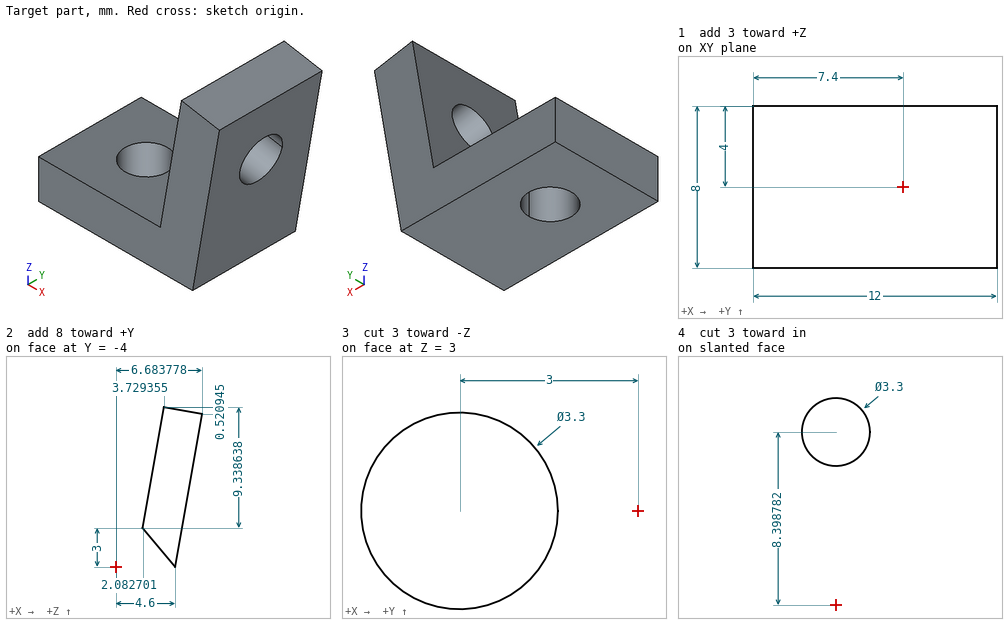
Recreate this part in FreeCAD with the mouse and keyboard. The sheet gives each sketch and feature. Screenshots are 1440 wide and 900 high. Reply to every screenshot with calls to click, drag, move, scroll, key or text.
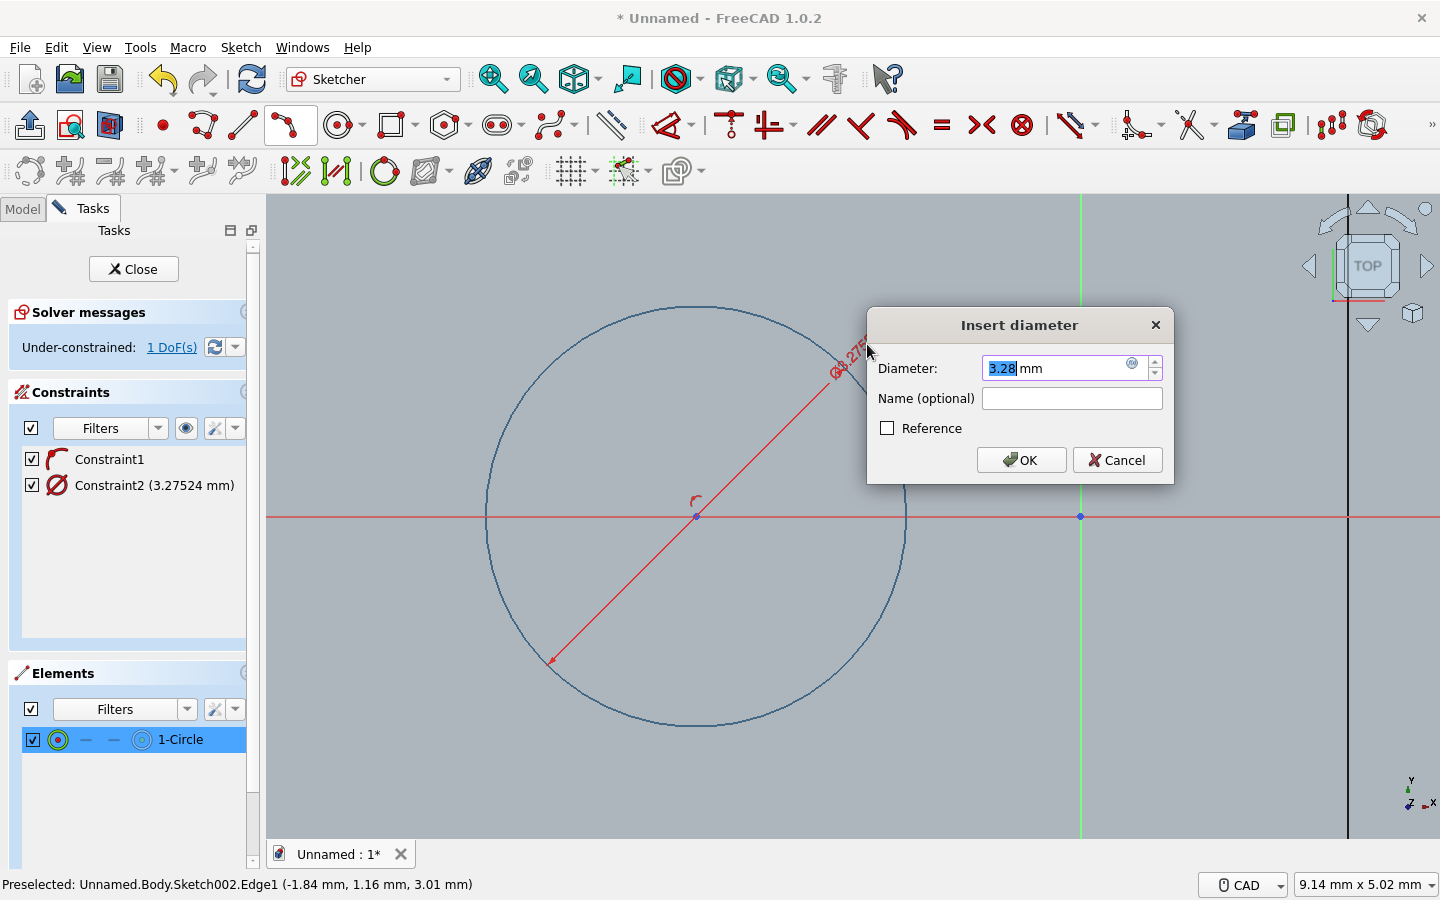
text(3.3)
key(Return)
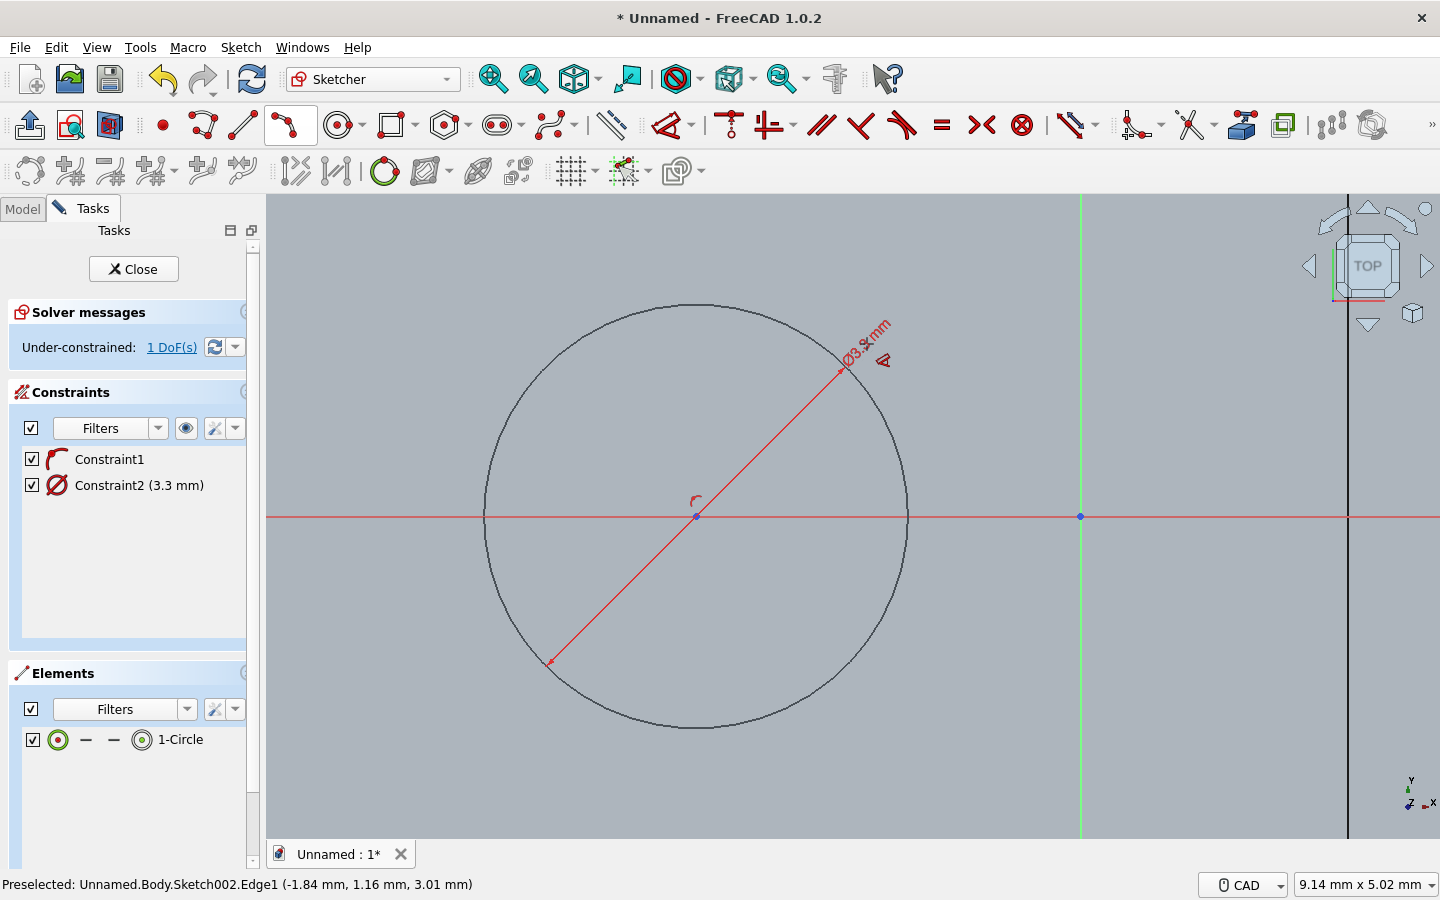
click(696, 516)
click(888, 550)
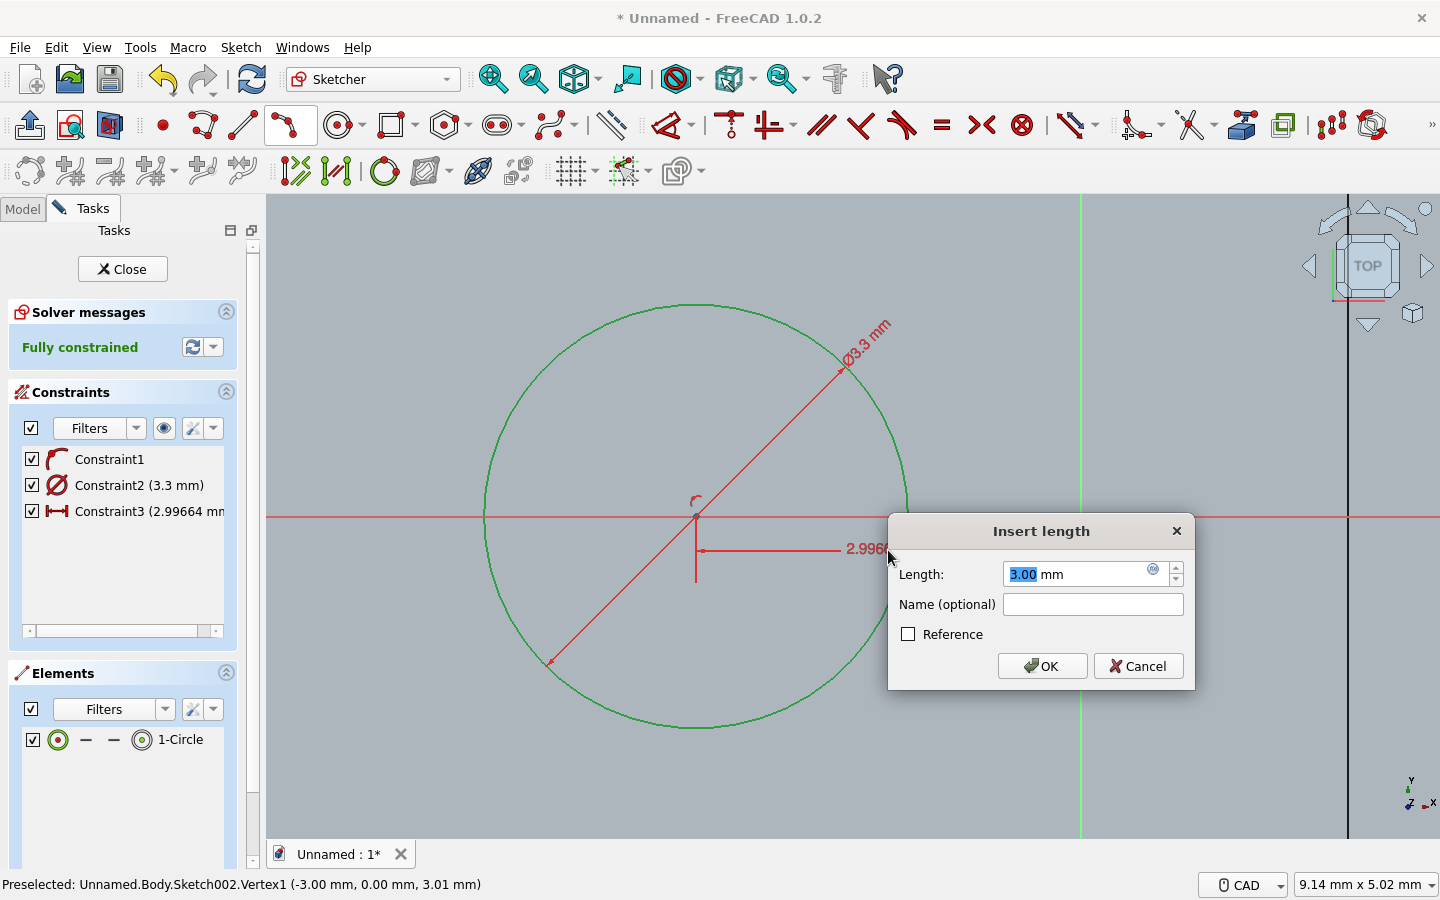
text(3)
key(Return)
key(Escape)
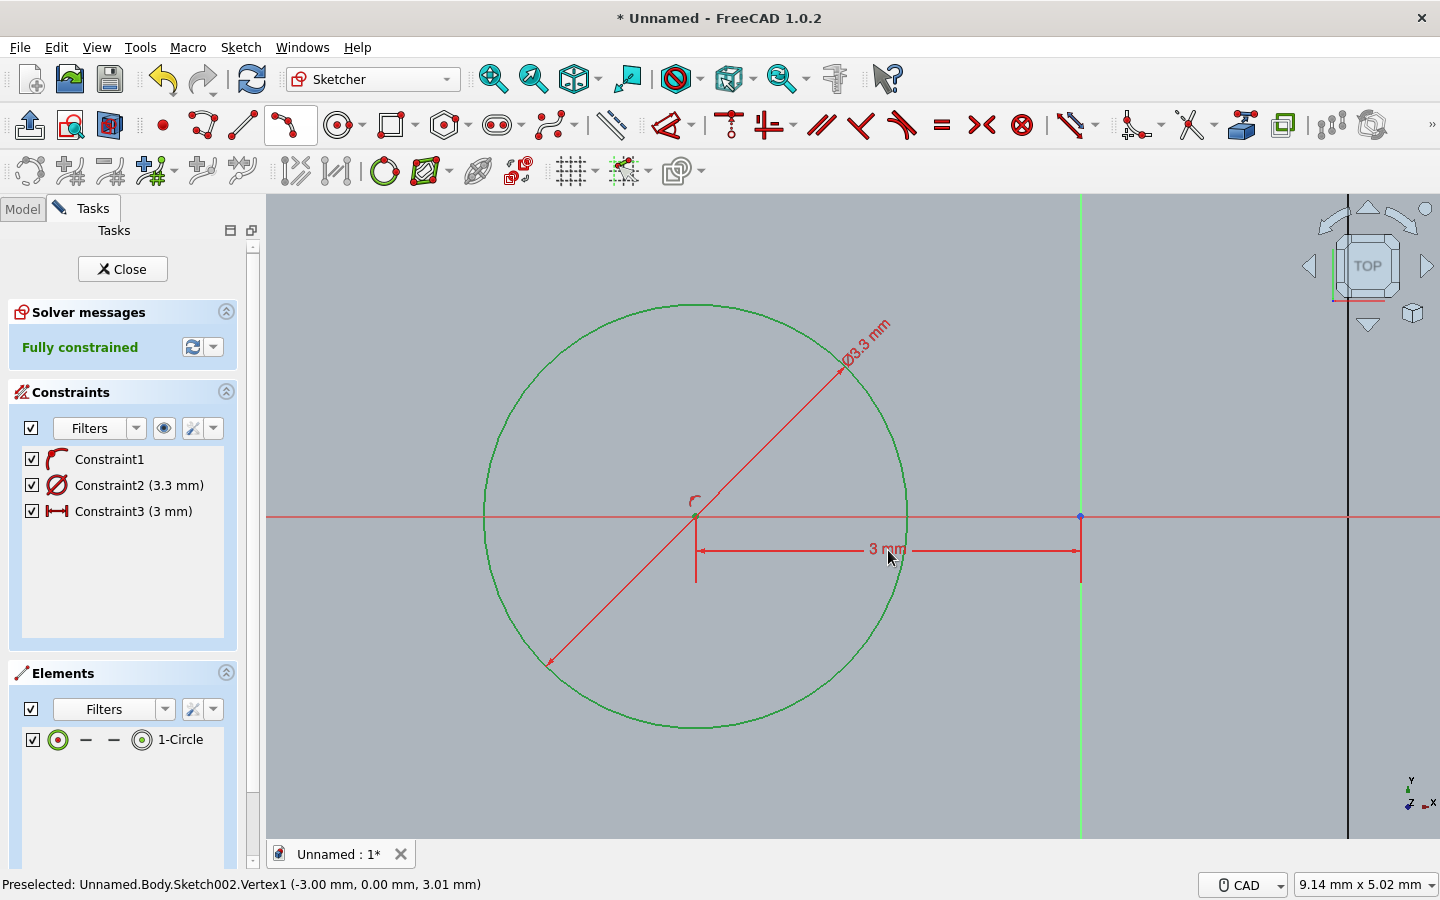
click(123, 269)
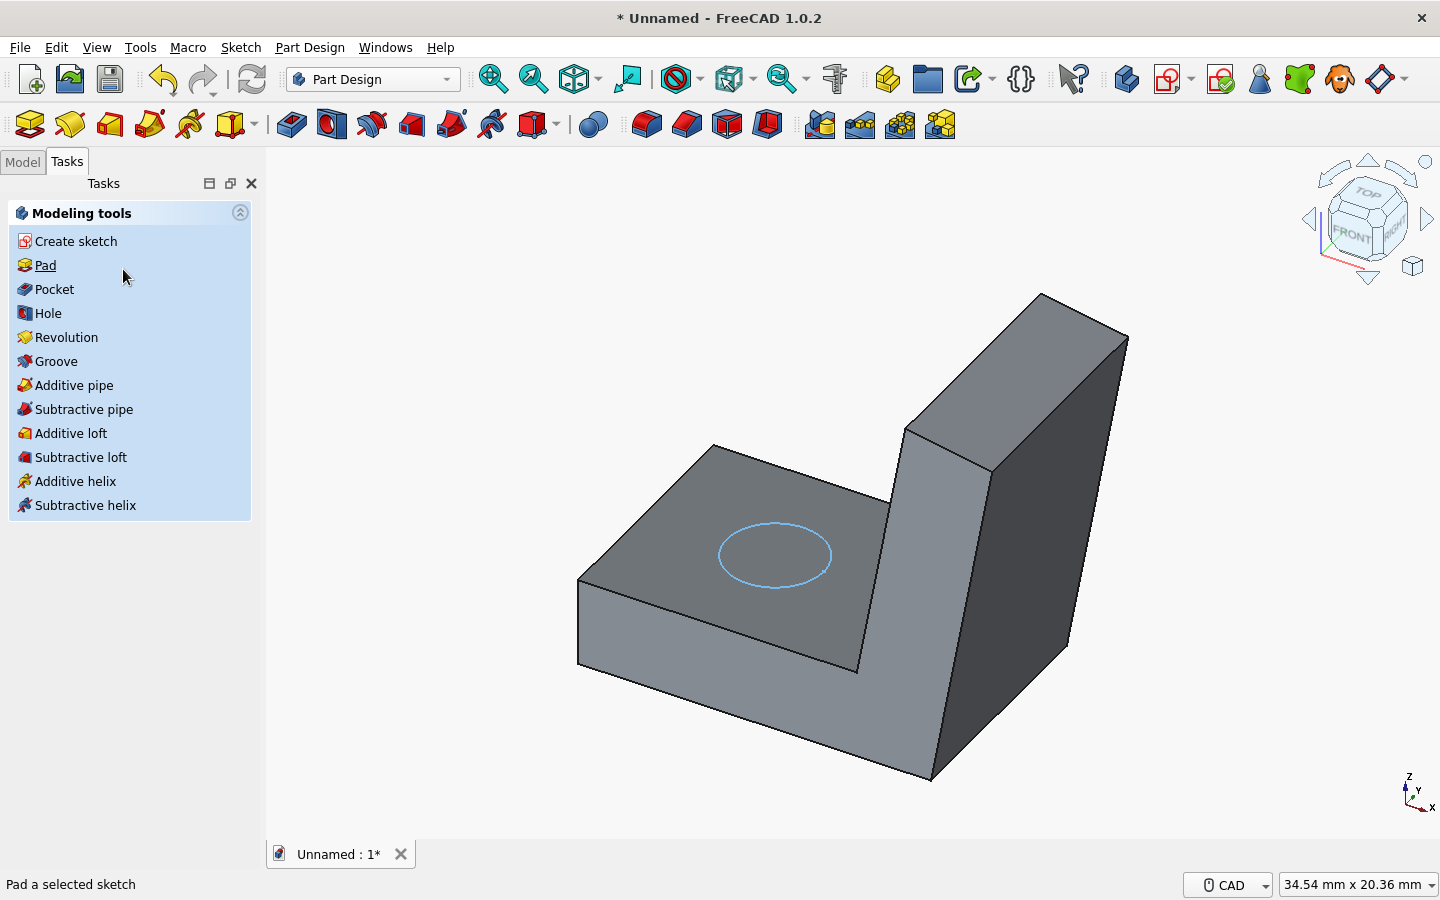
click(292, 124)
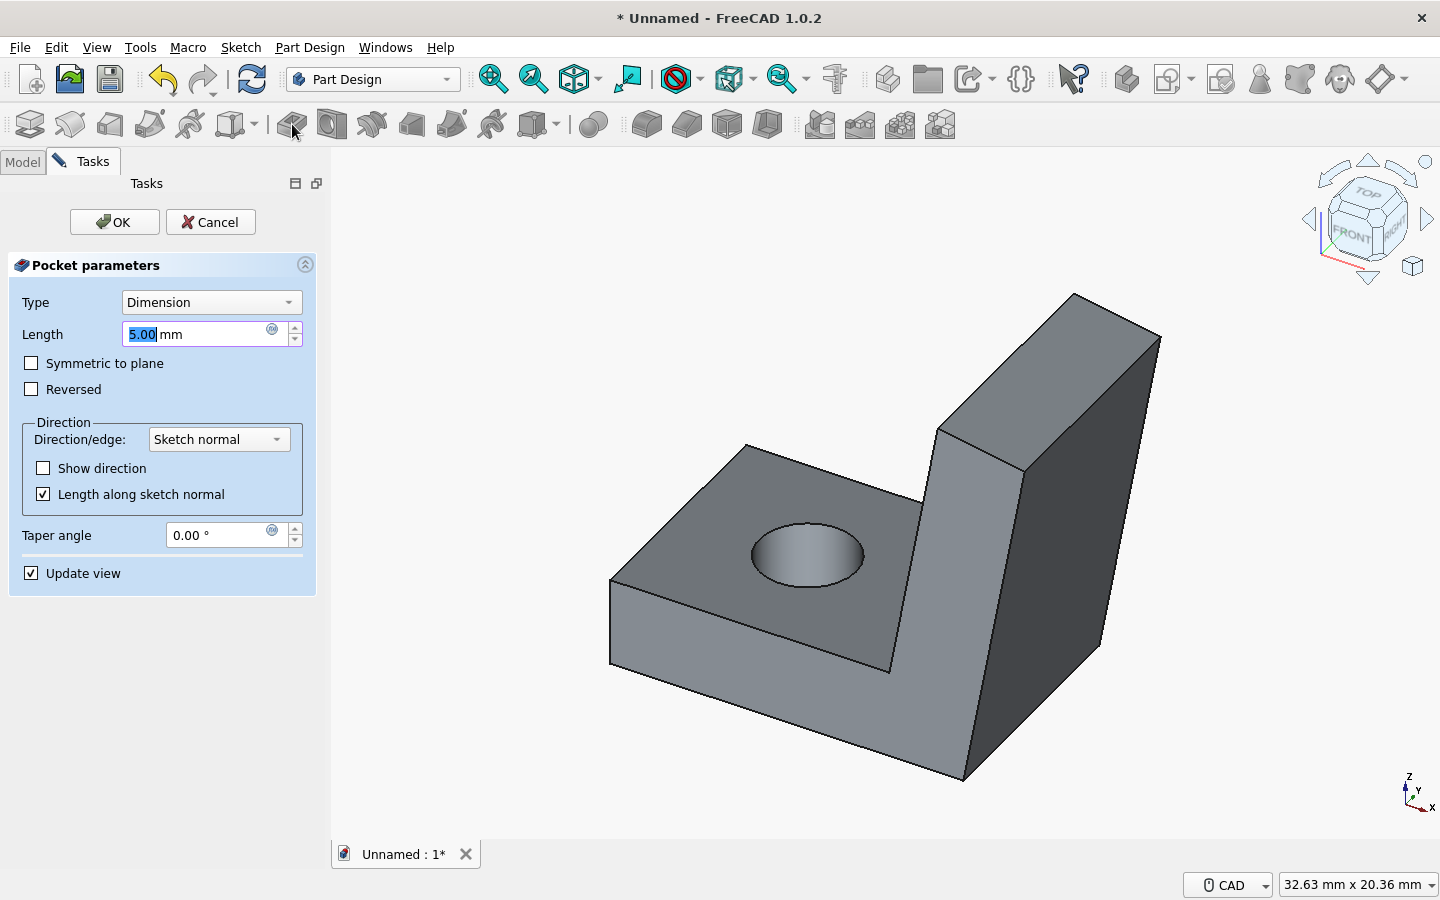
text(3)
key(Tab)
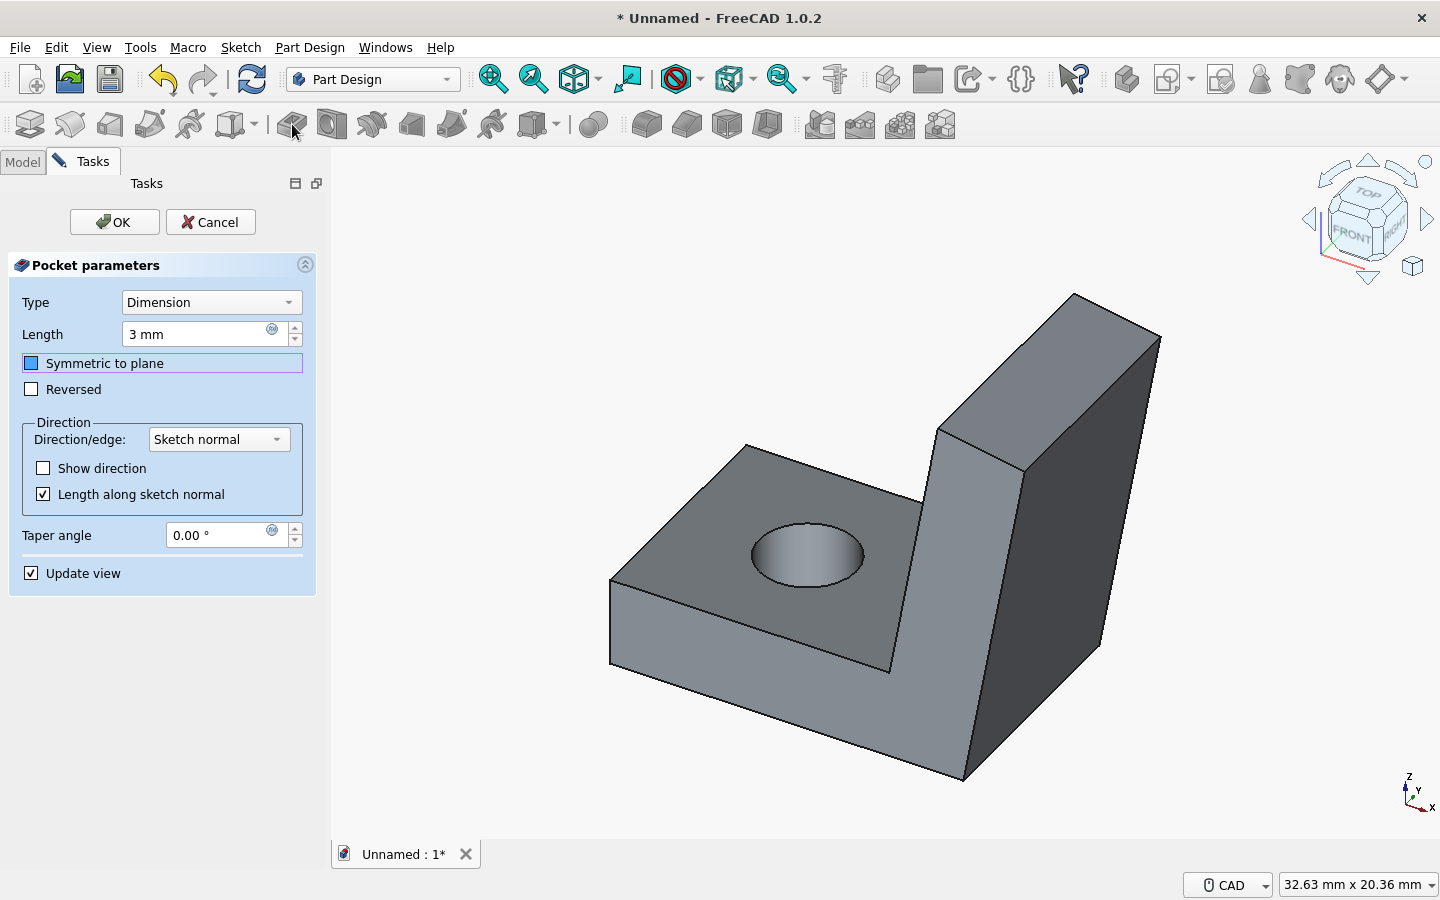
click(115, 222)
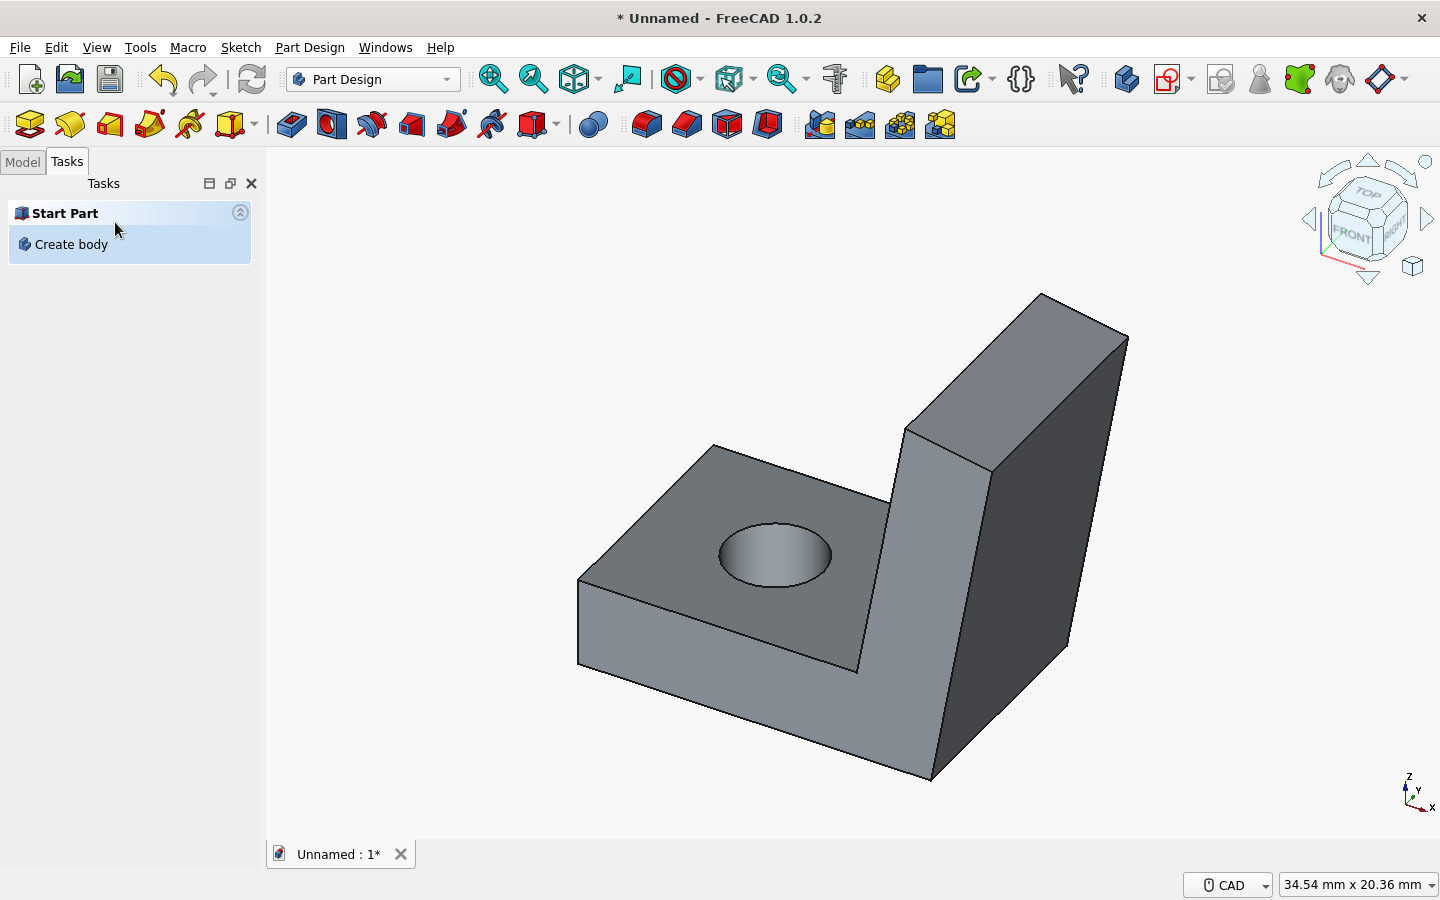
click(1038, 514)